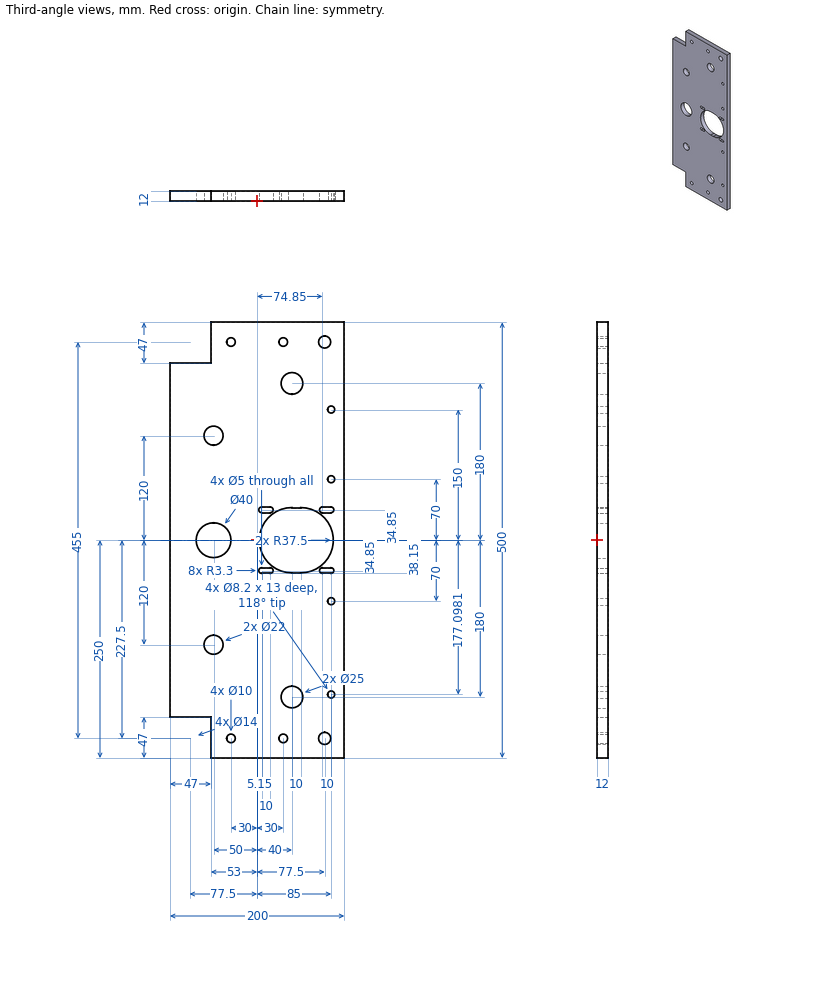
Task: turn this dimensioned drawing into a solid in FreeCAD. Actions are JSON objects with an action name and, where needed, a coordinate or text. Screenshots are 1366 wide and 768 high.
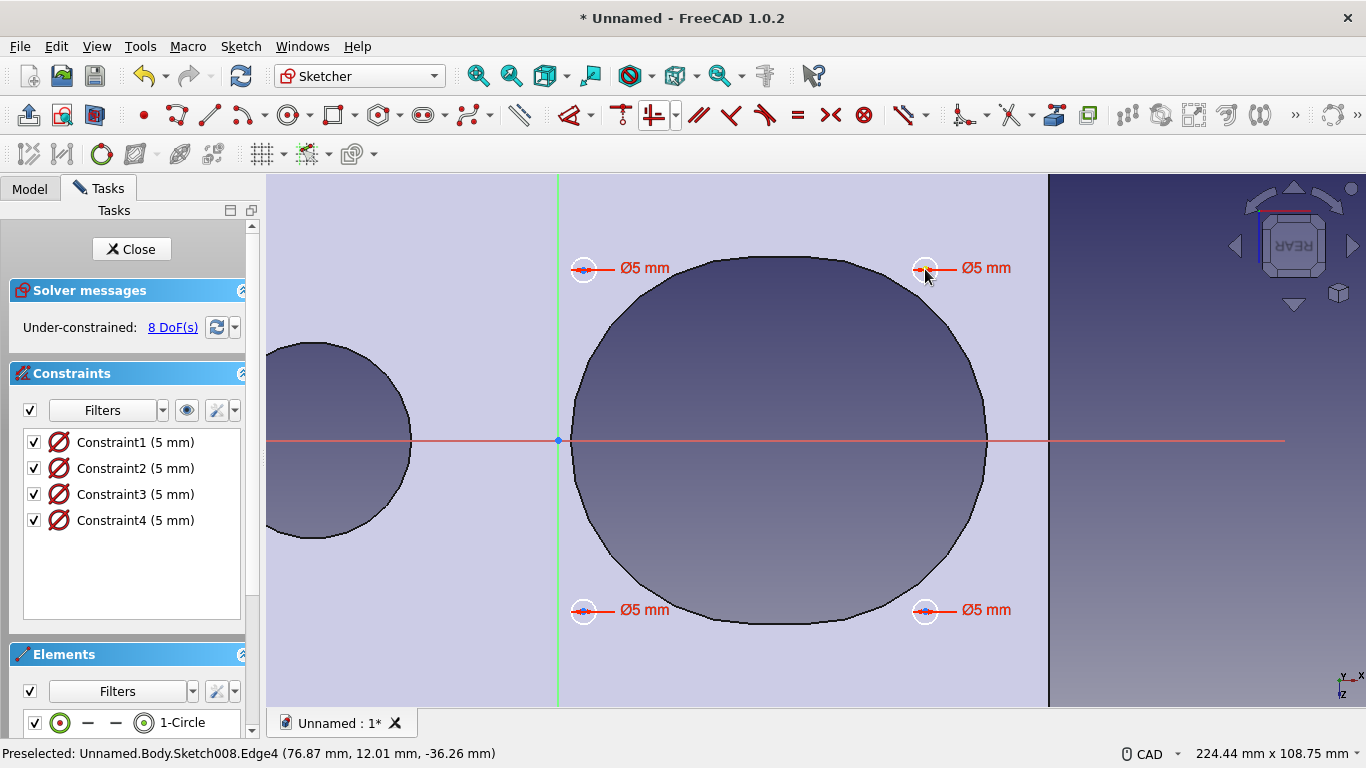
{"action": "left_click", "coordinate": [584, 270]}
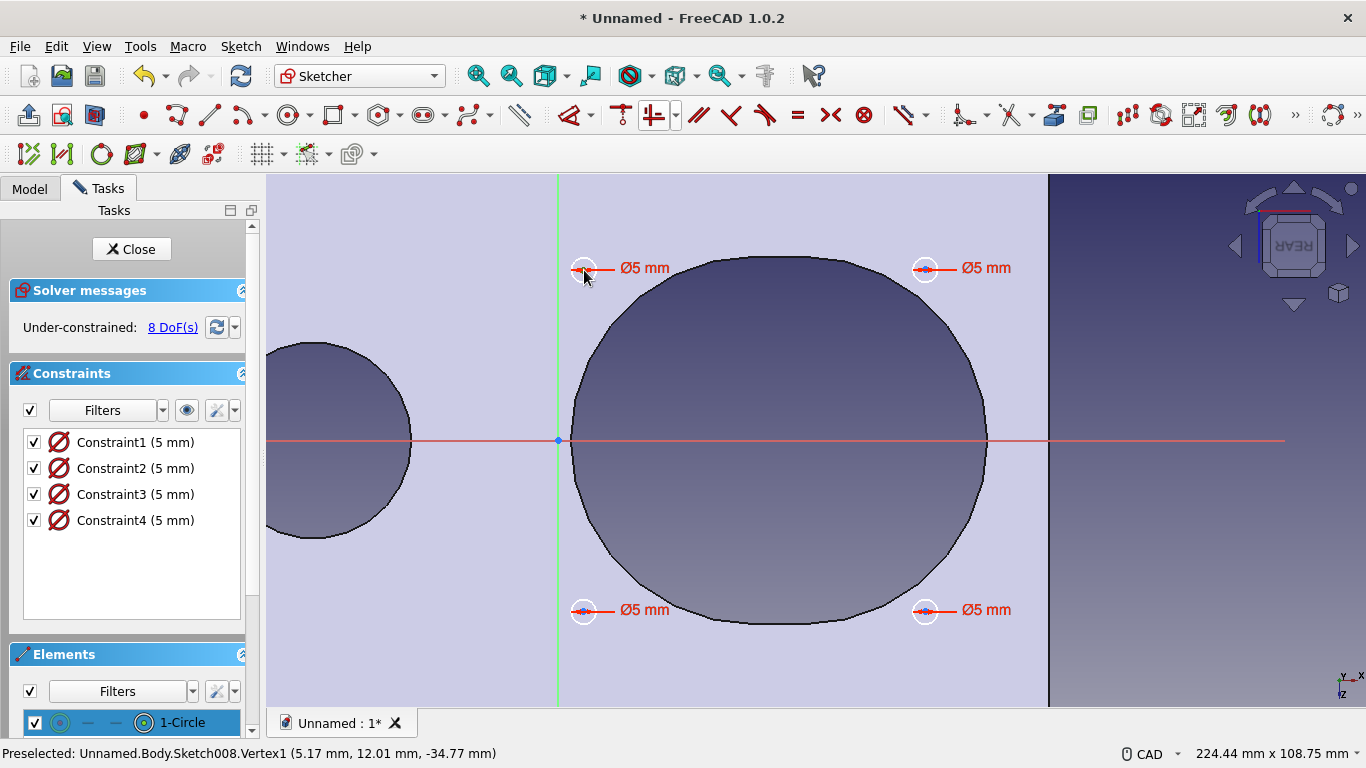
{"action": "left_click", "coordinate": [584, 612]}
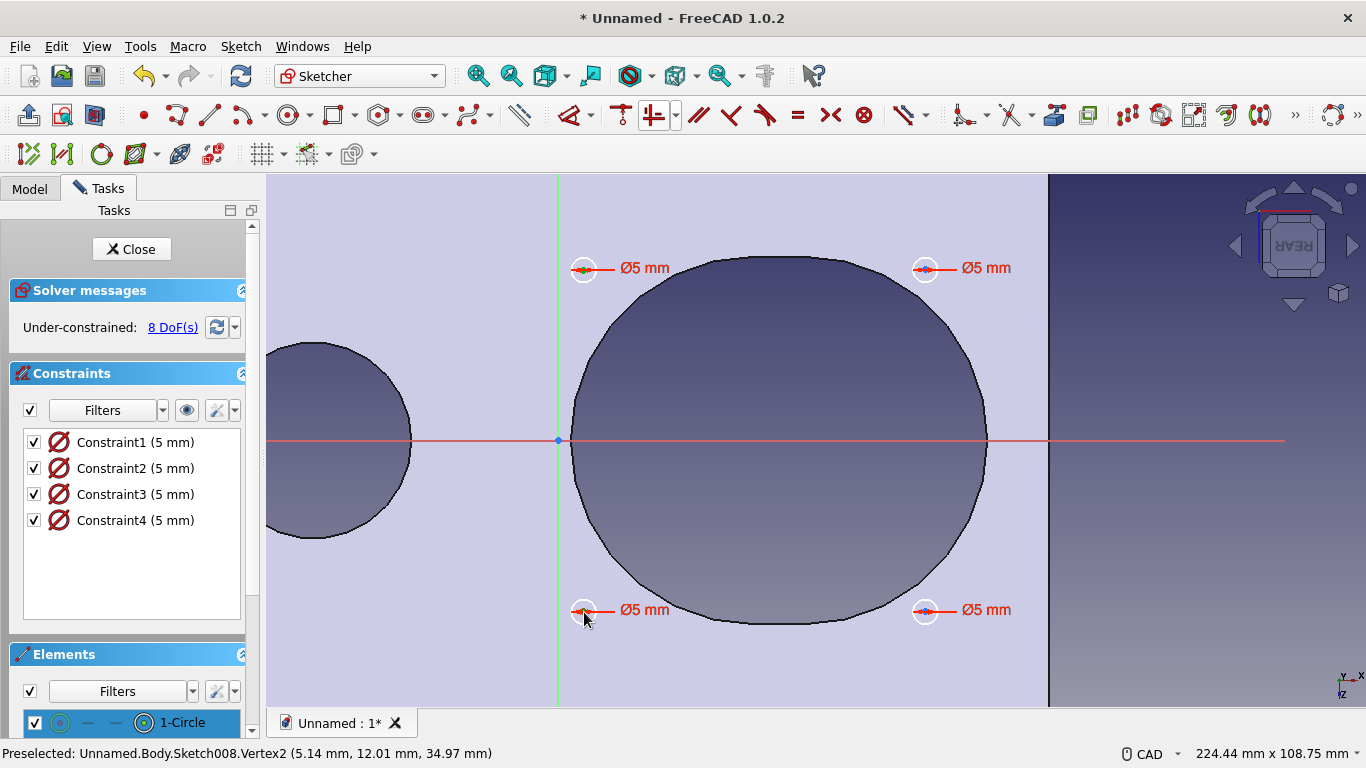
{"action": "key", "text": "v"}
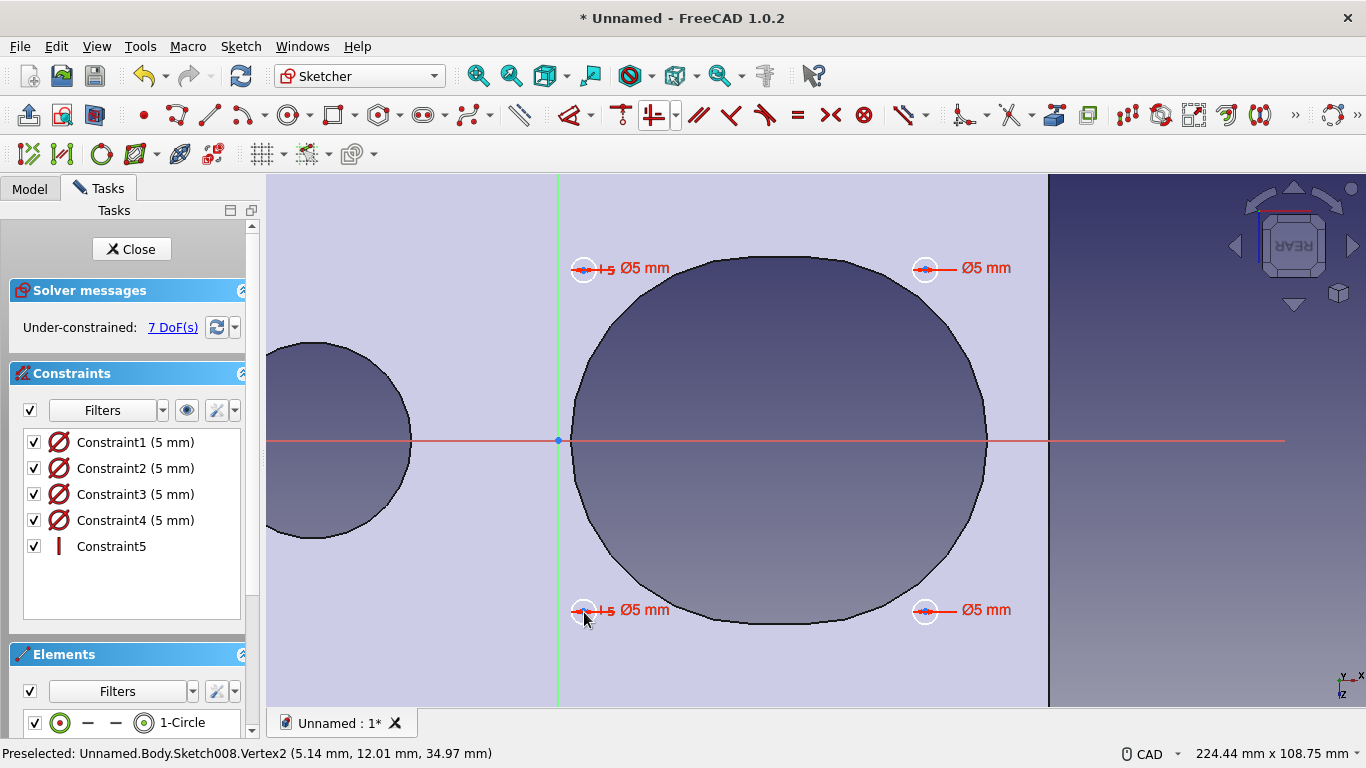
{"action": "left_click", "coordinate": [584, 612]}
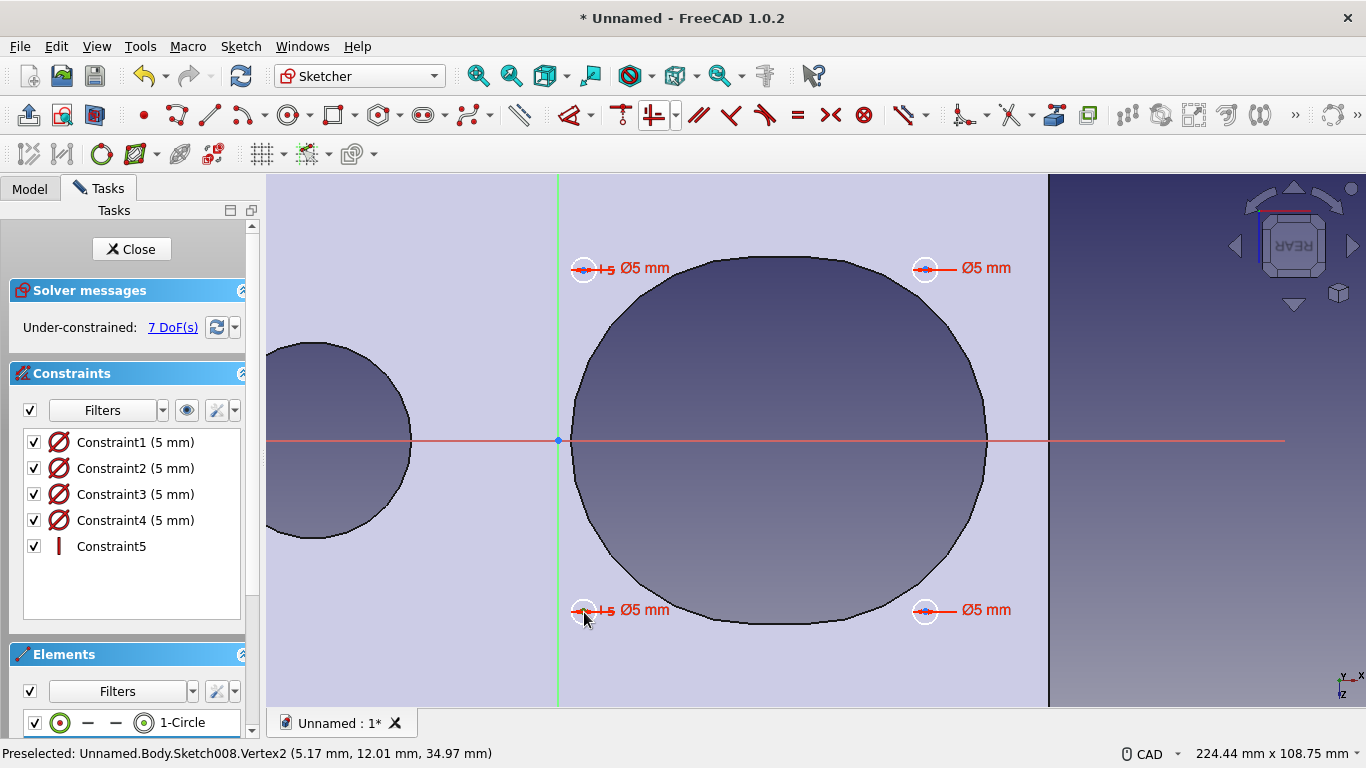
{"action": "left_click", "coordinate": [925, 612]}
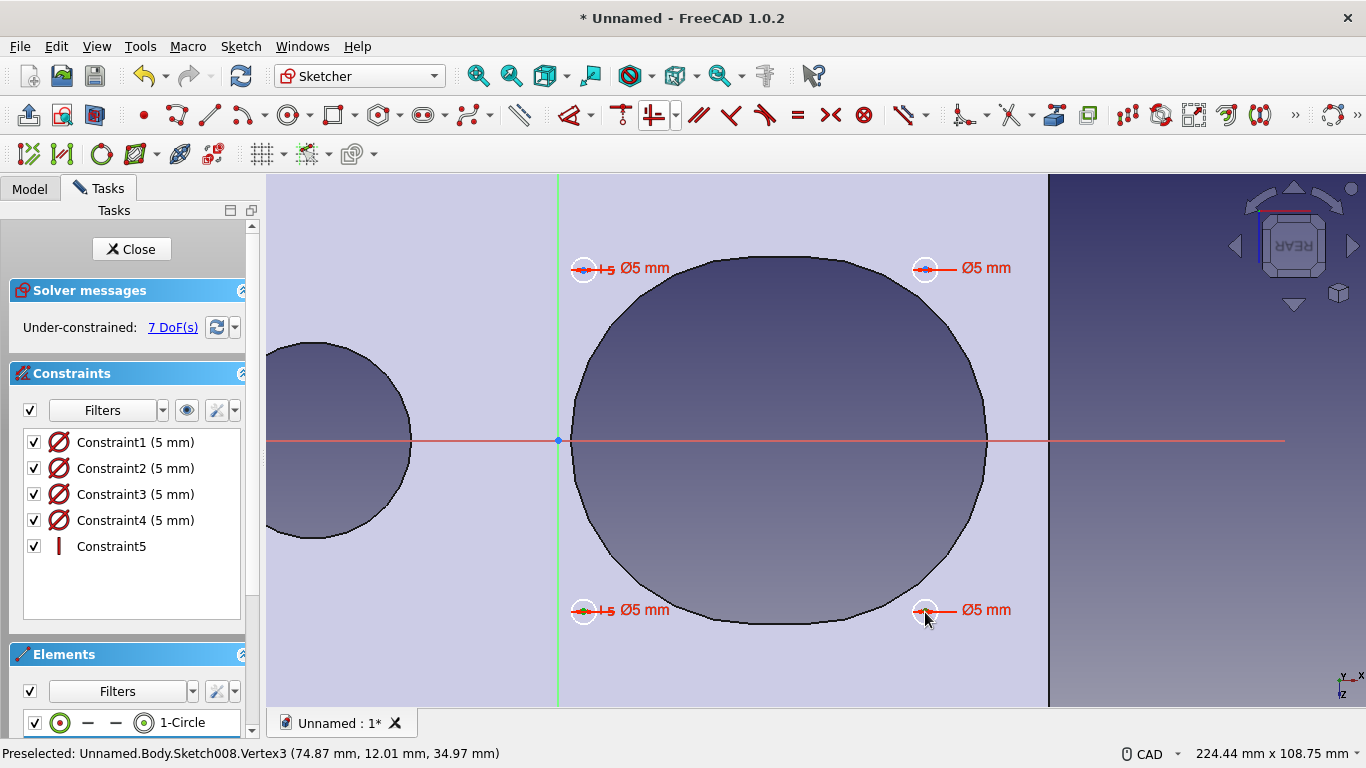
{"action": "left_click", "coordinate": [676, 116]}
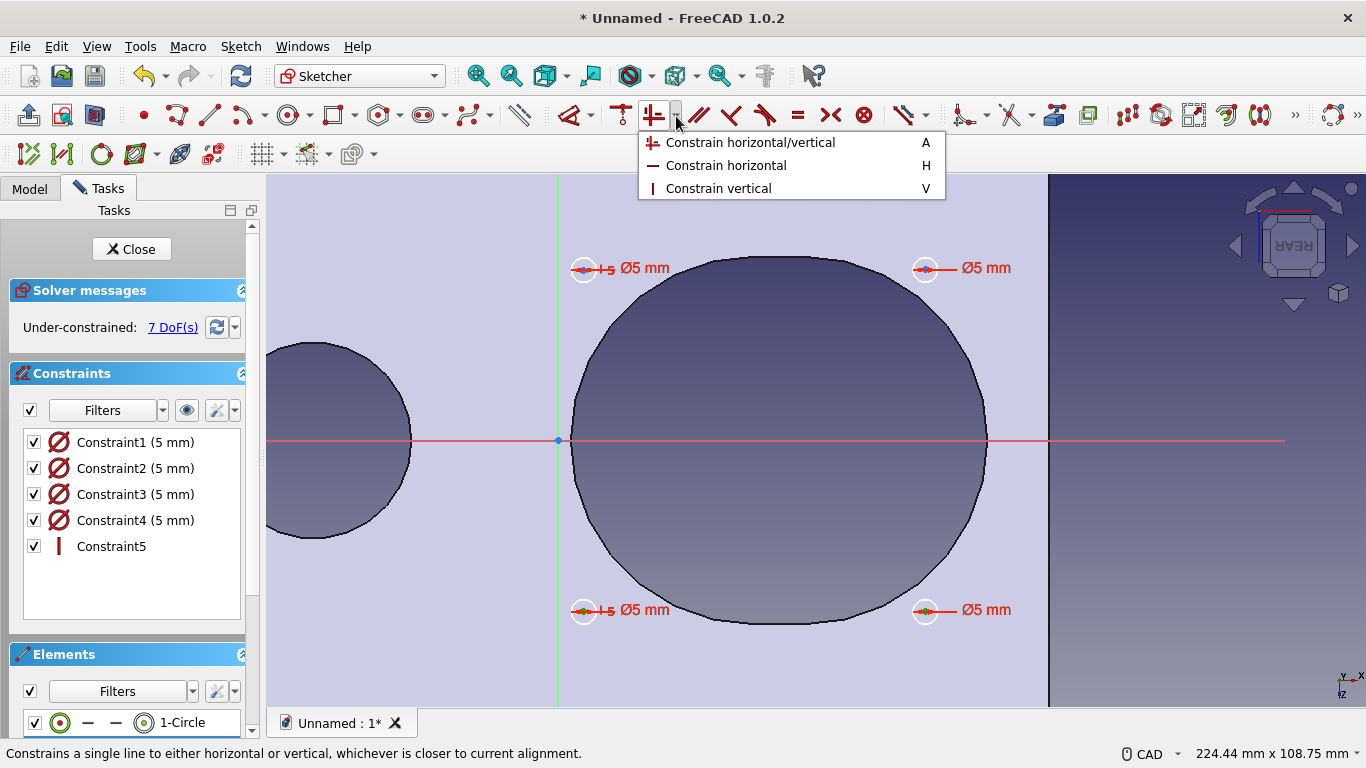
{"action": "left_click", "coordinate": [792, 166]}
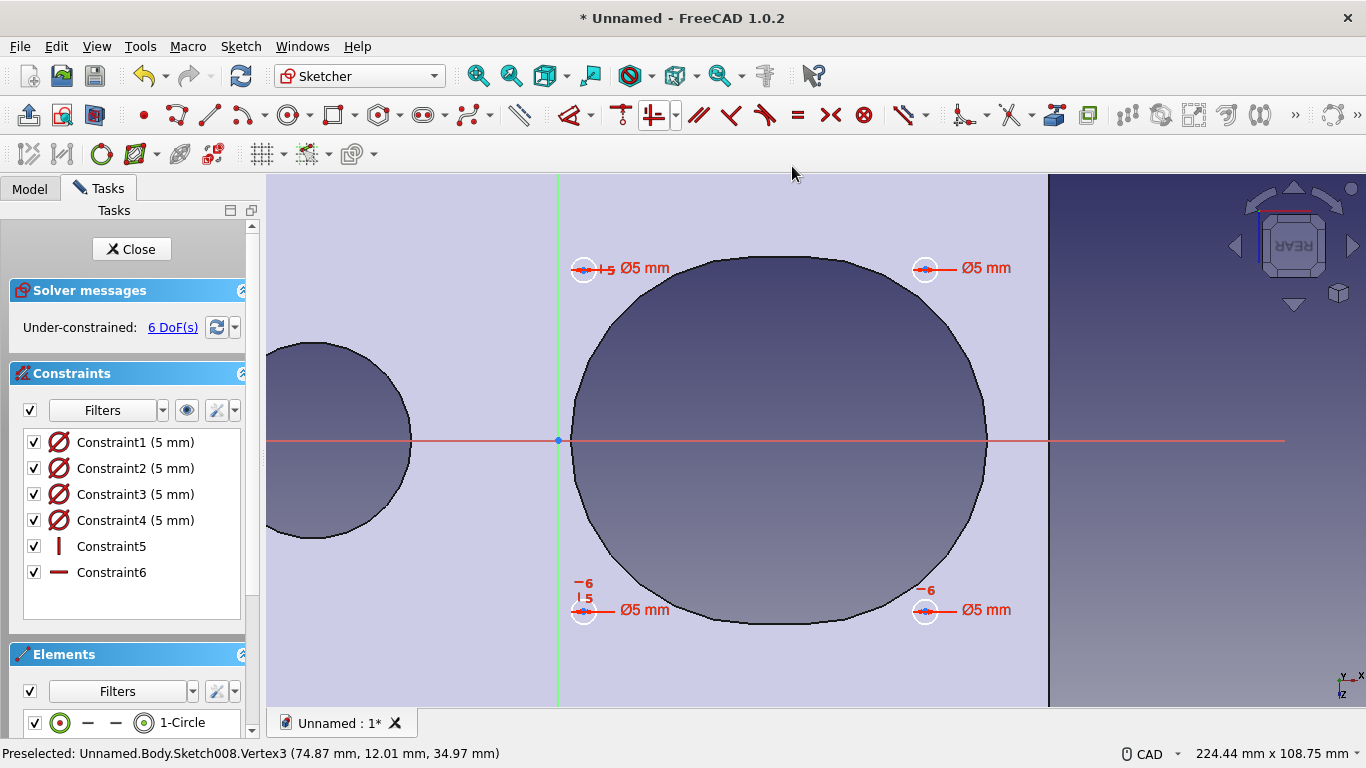
{"action": "left_click", "coordinate": [925, 612]}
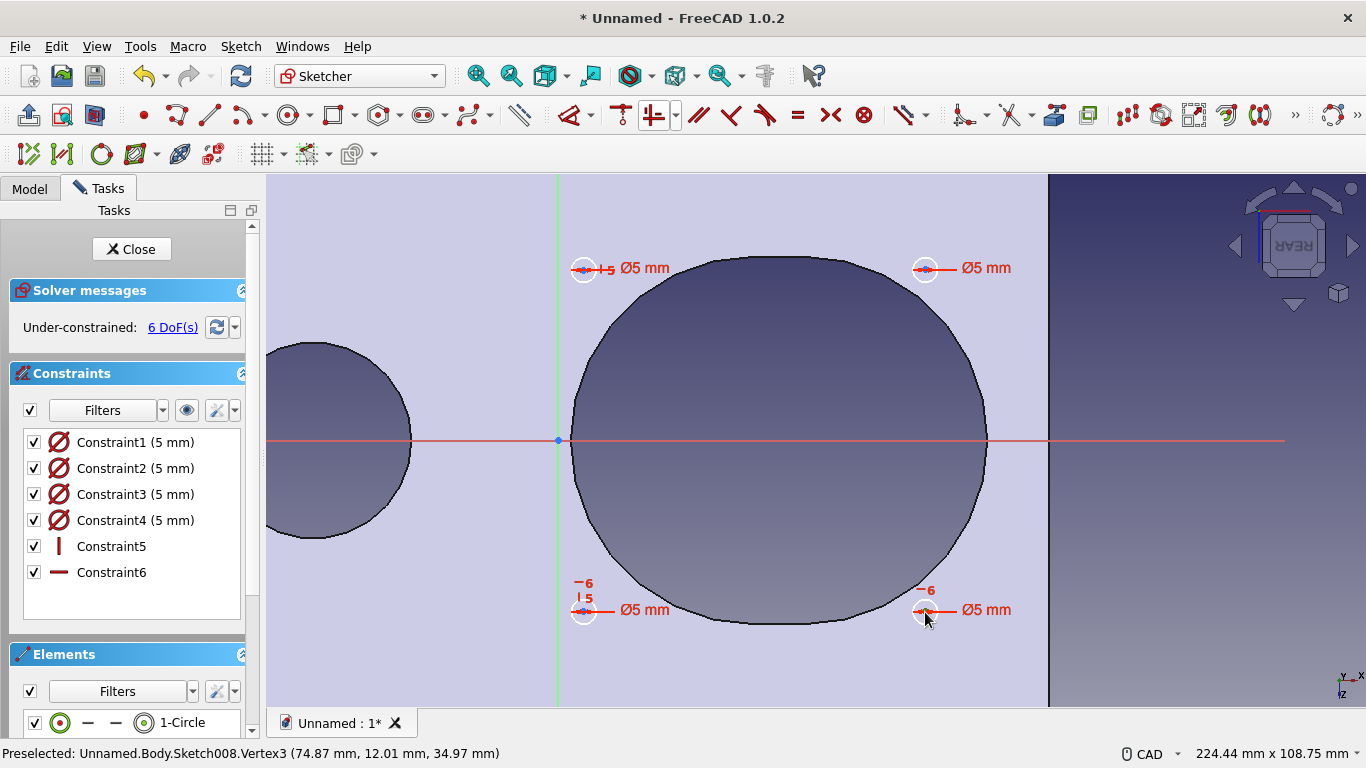
{"action": "left_click", "coordinate": [925, 270]}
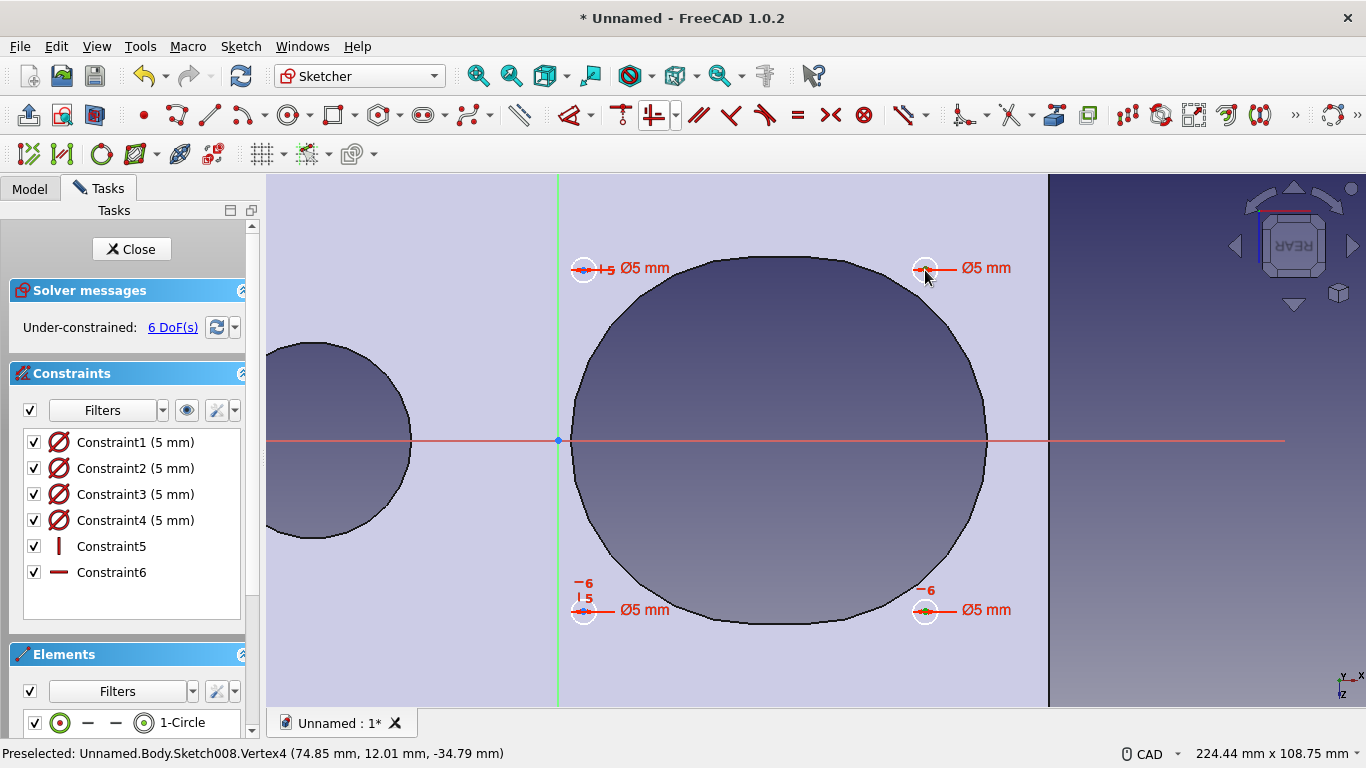
{"action": "key", "text": "v"}